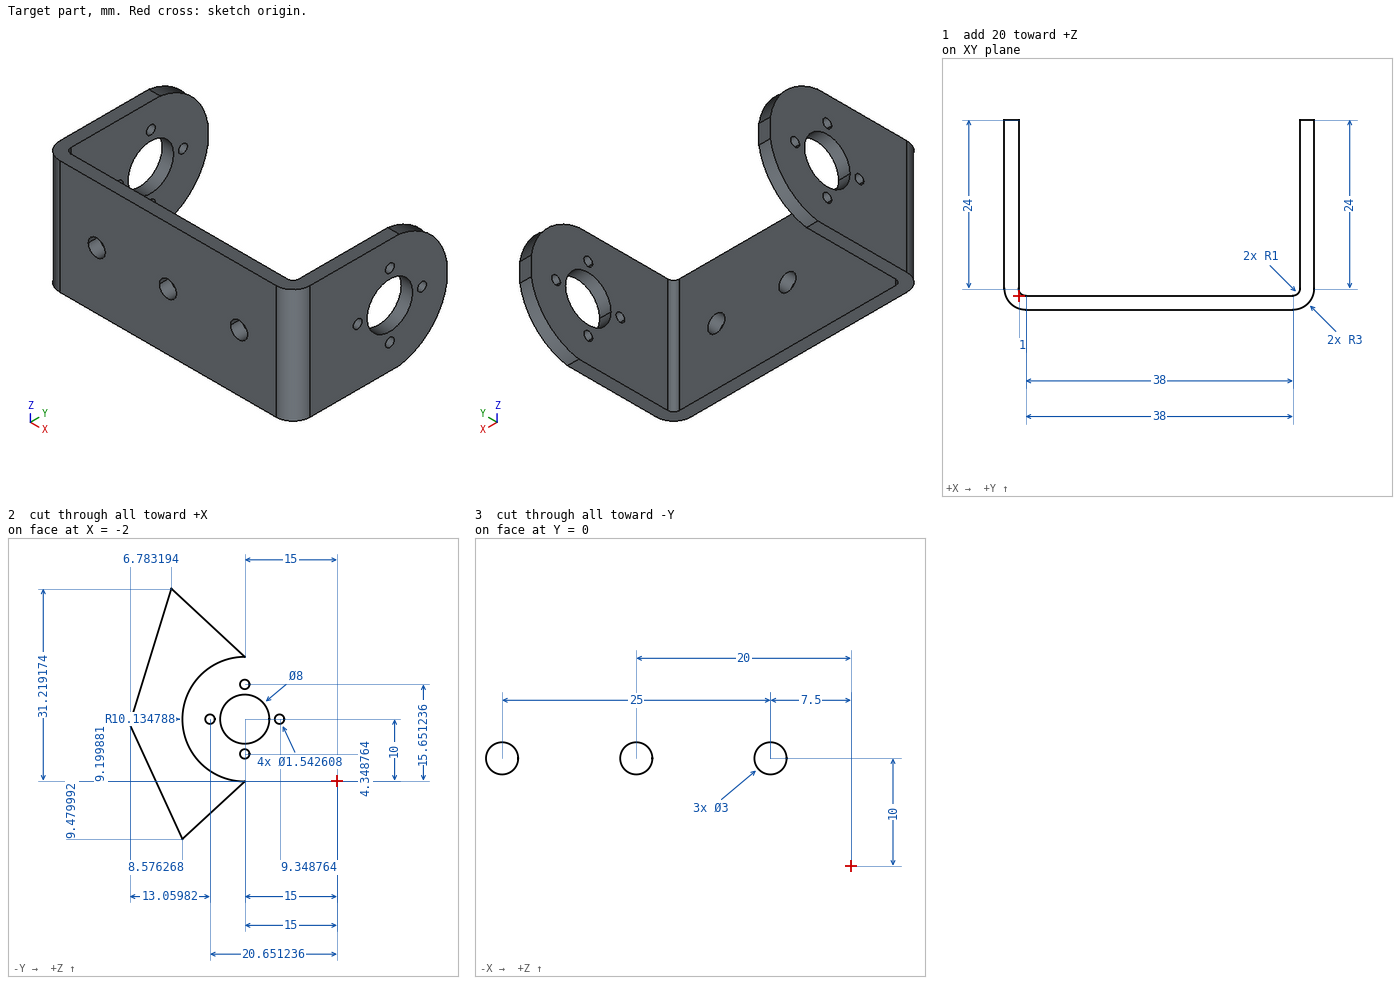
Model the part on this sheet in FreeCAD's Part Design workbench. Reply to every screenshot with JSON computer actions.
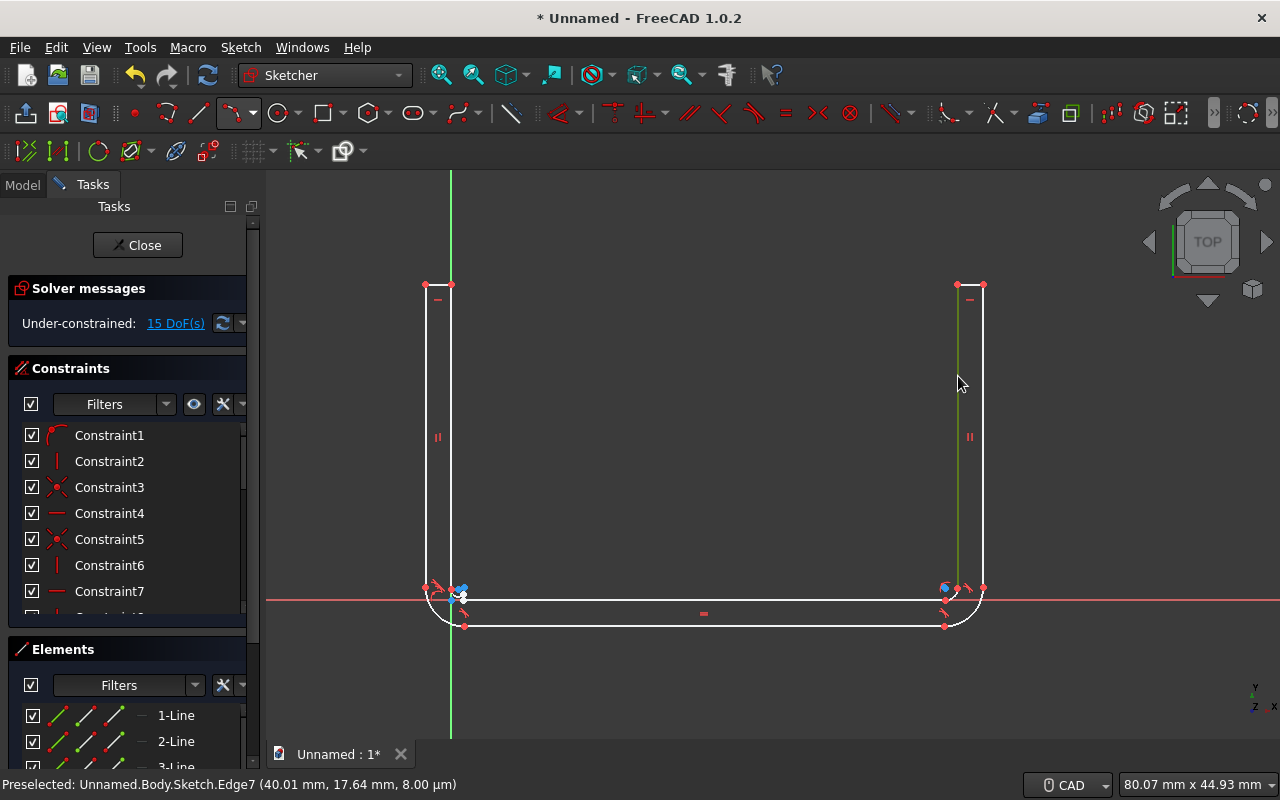
{"action": "scroll", "coordinate": [954, 597], "scroll_direction": "up", "scroll_amount": 2}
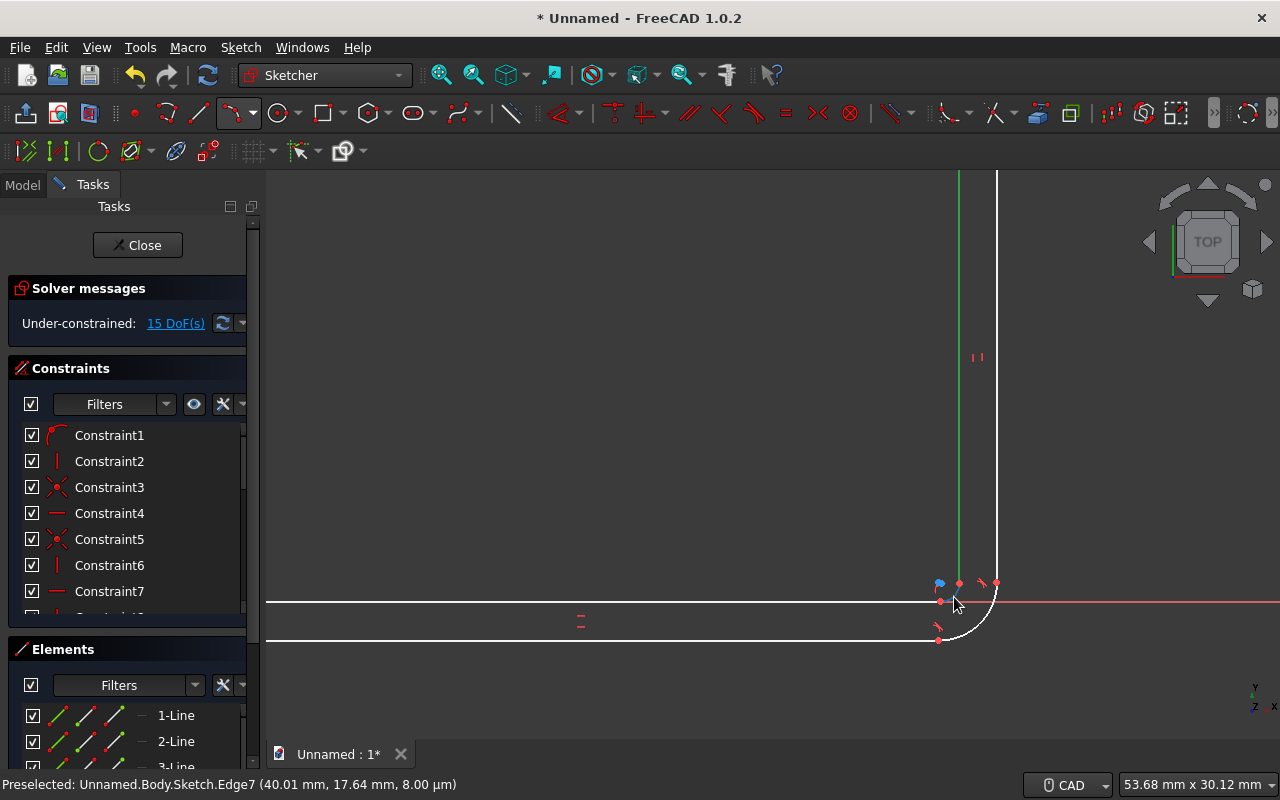
{"action": "left_click", "coordinate": [954, 597]}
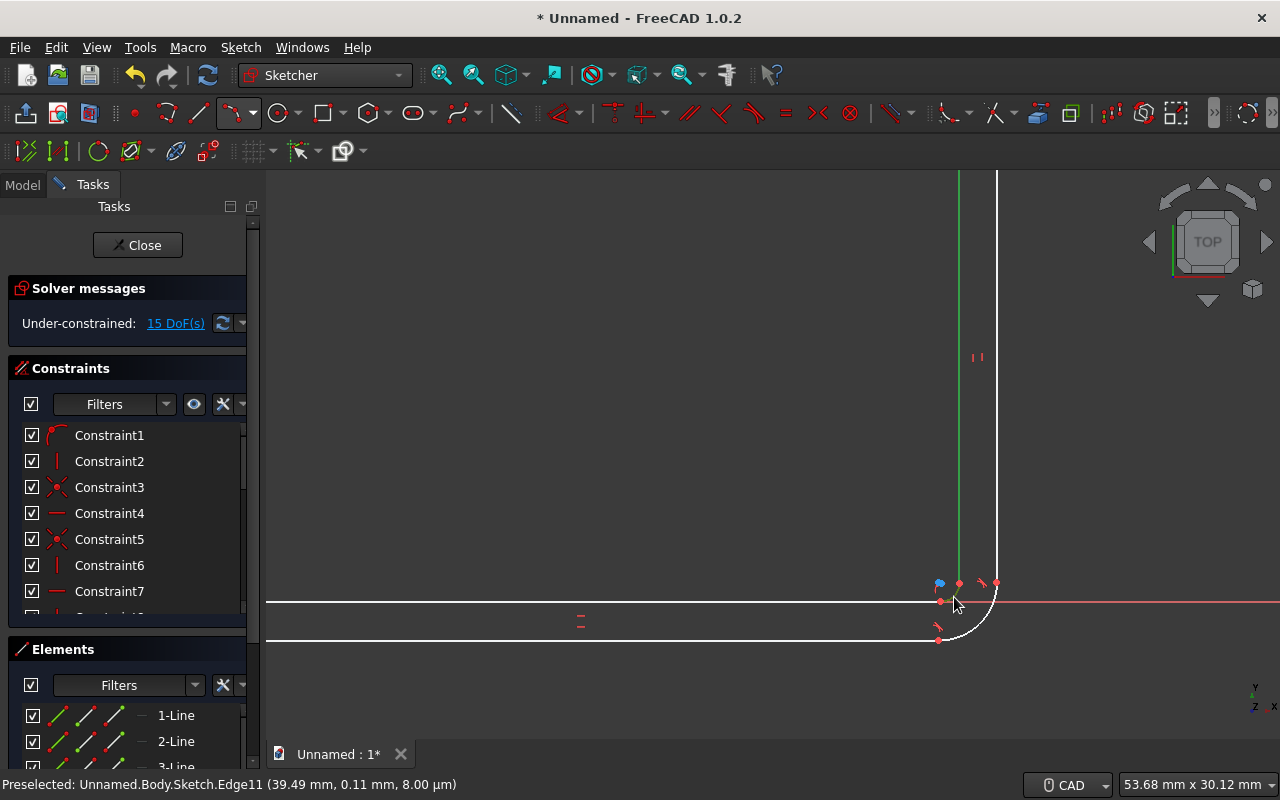
{"action": "left_click", "coordinate": [754, 114]}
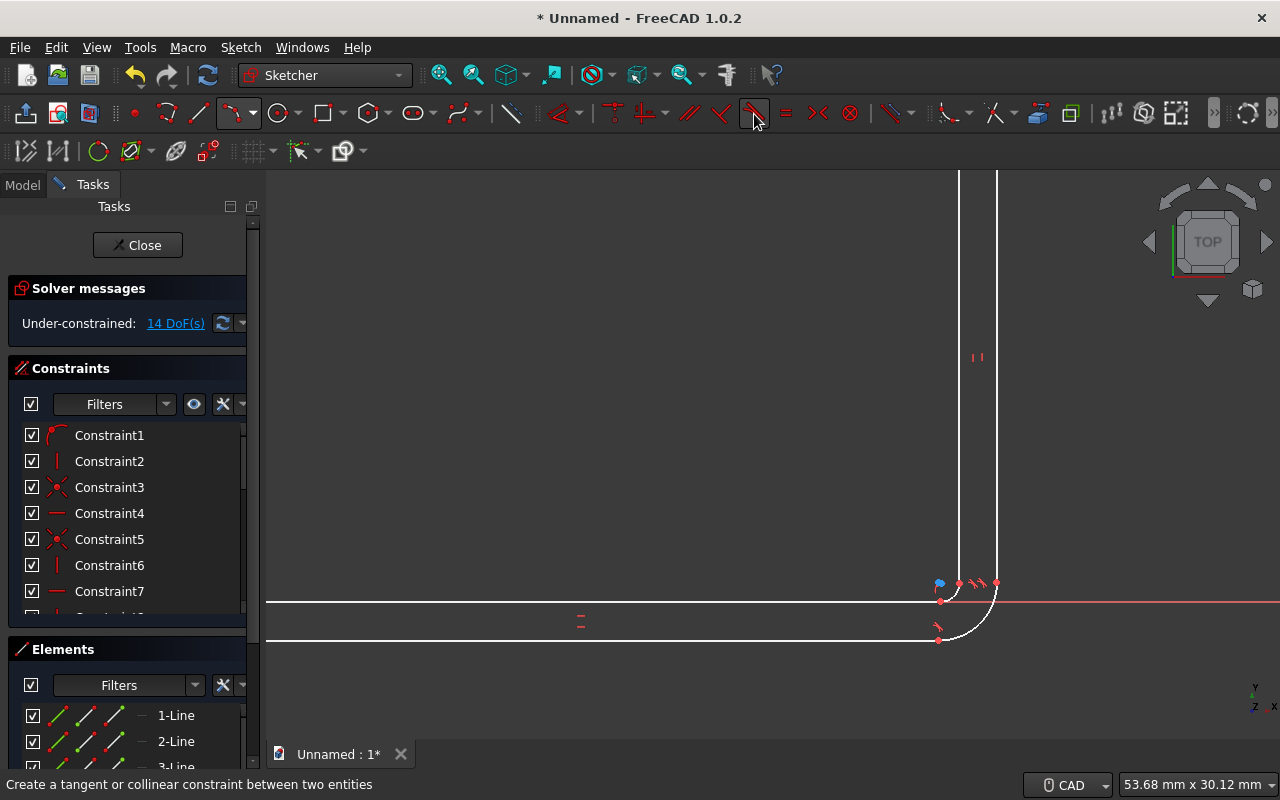
{"action": "left_click", "coordinate": [725, 602]}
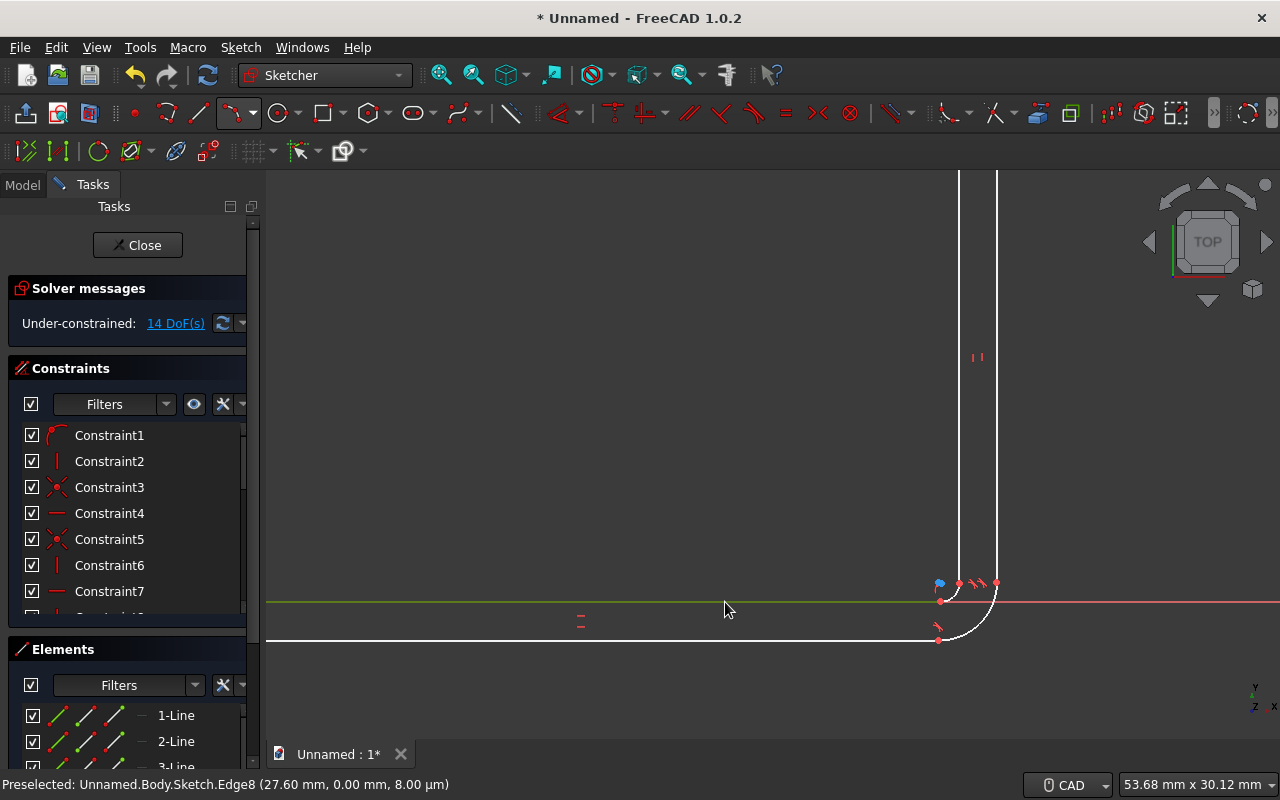
{"action": "scroll", "coordinate": [949, 600], "scroll_direction": "up", "scroll_amount": 3}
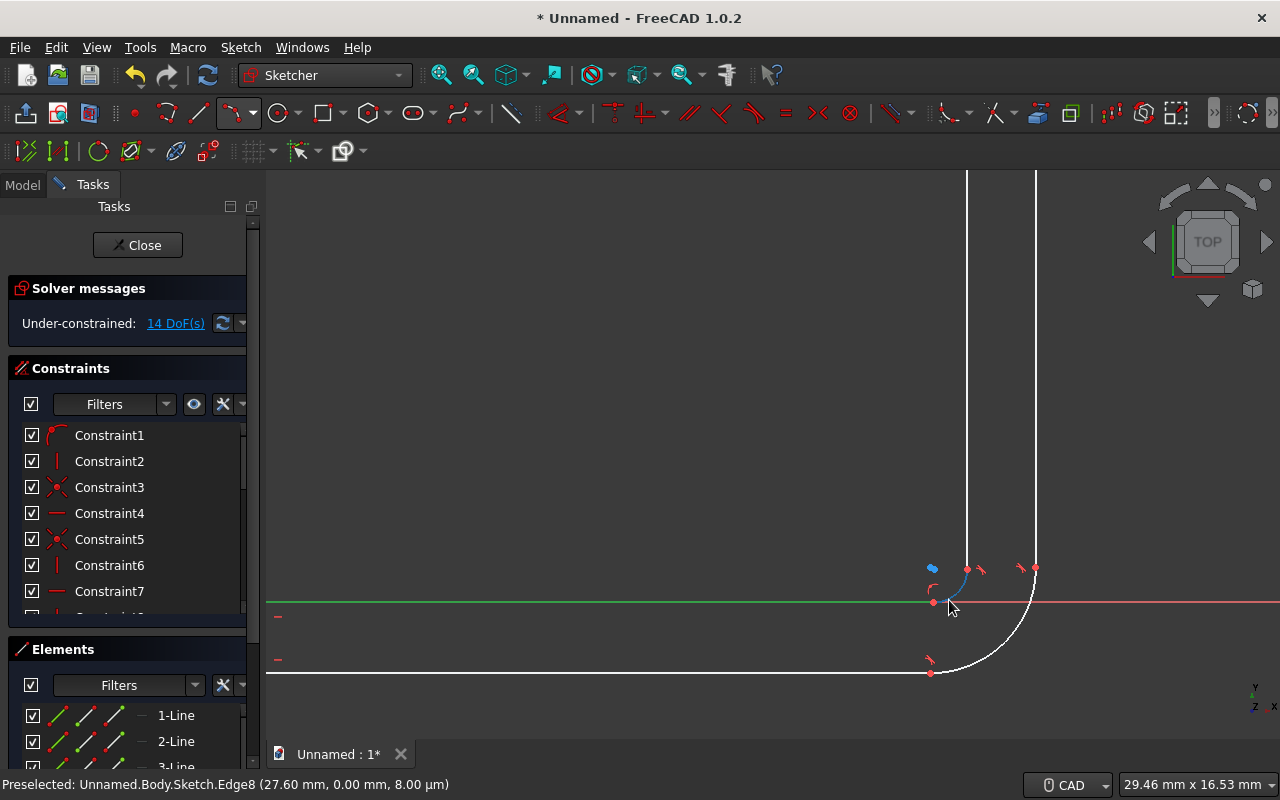
{"action": "left_click", "coordinate": [949, 599]}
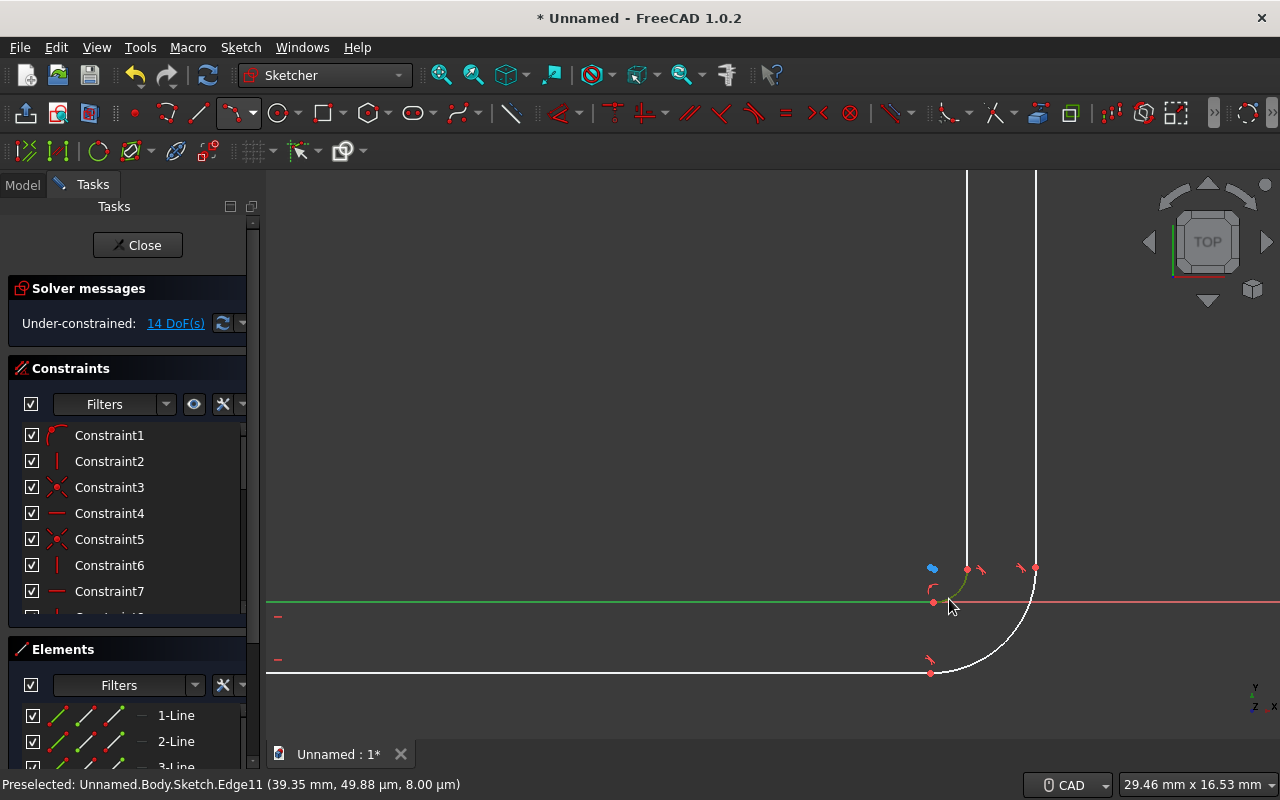
{"action": "left_click", "coordinate": [754, 114]}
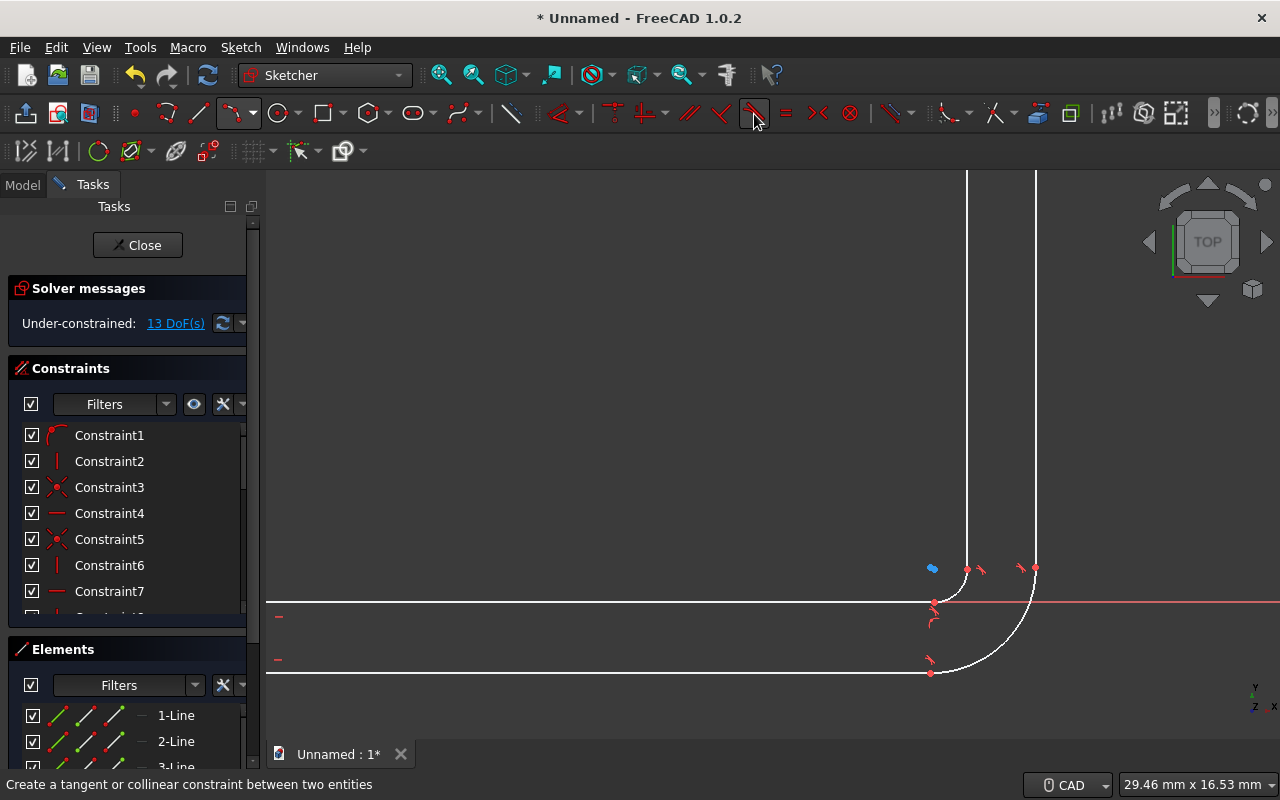
{"action": "left_click", "coordinate": [541, 602]}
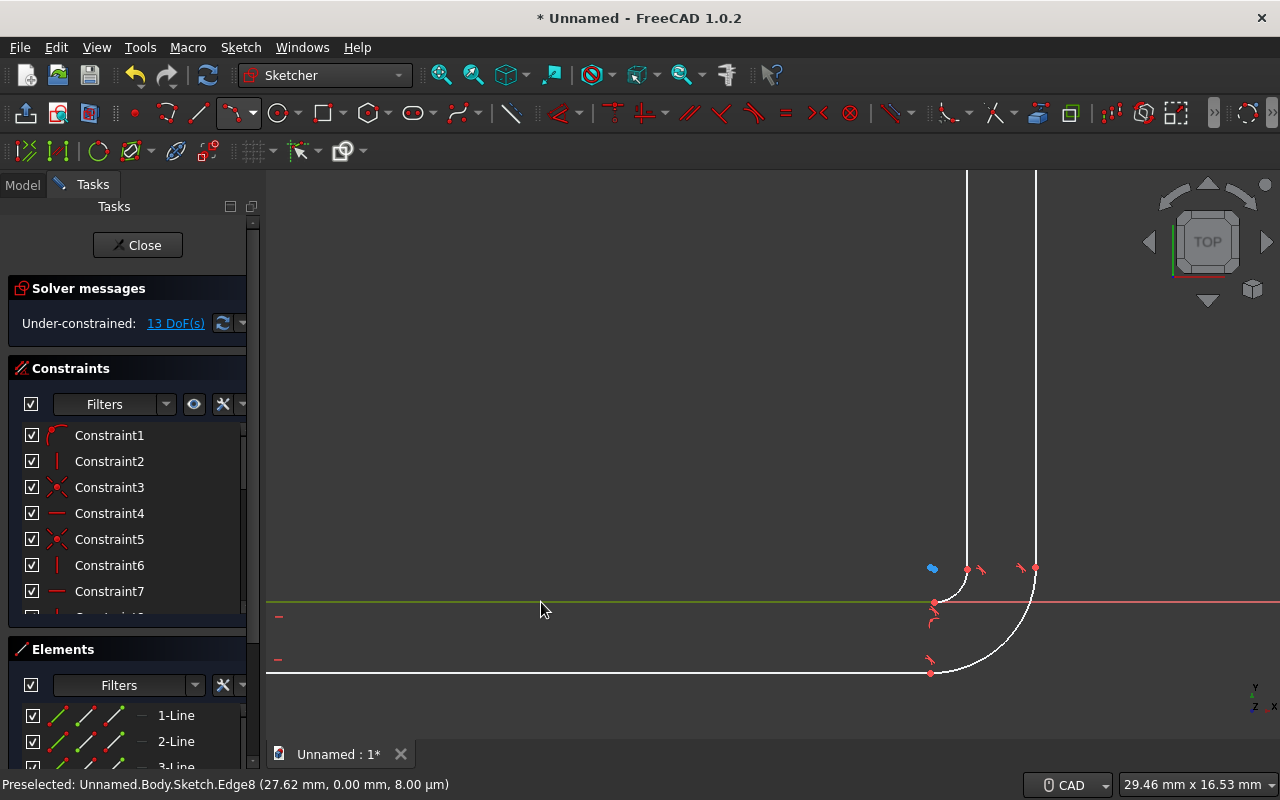
{"action": "scroll", "coordinate": [952, 599], "scroll_direction": "down", "scroll_amount": 5}